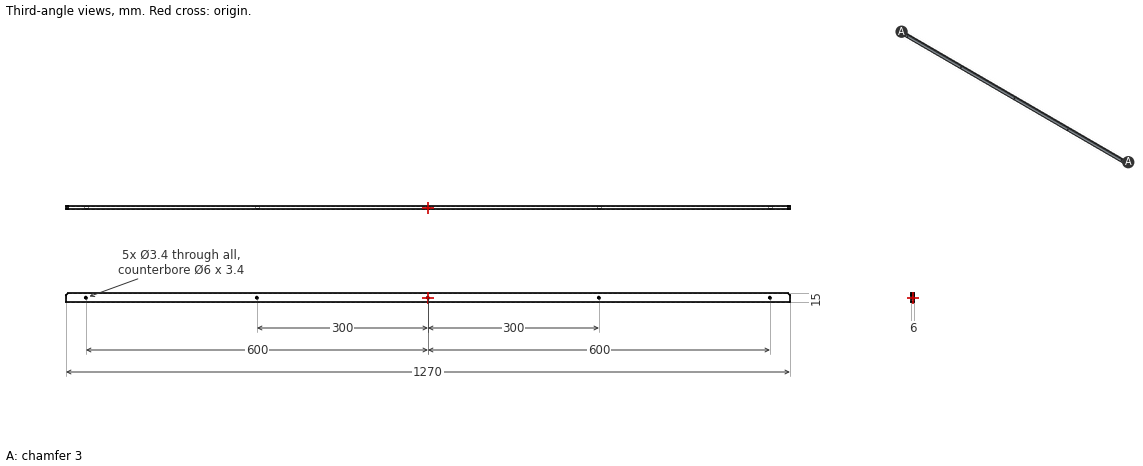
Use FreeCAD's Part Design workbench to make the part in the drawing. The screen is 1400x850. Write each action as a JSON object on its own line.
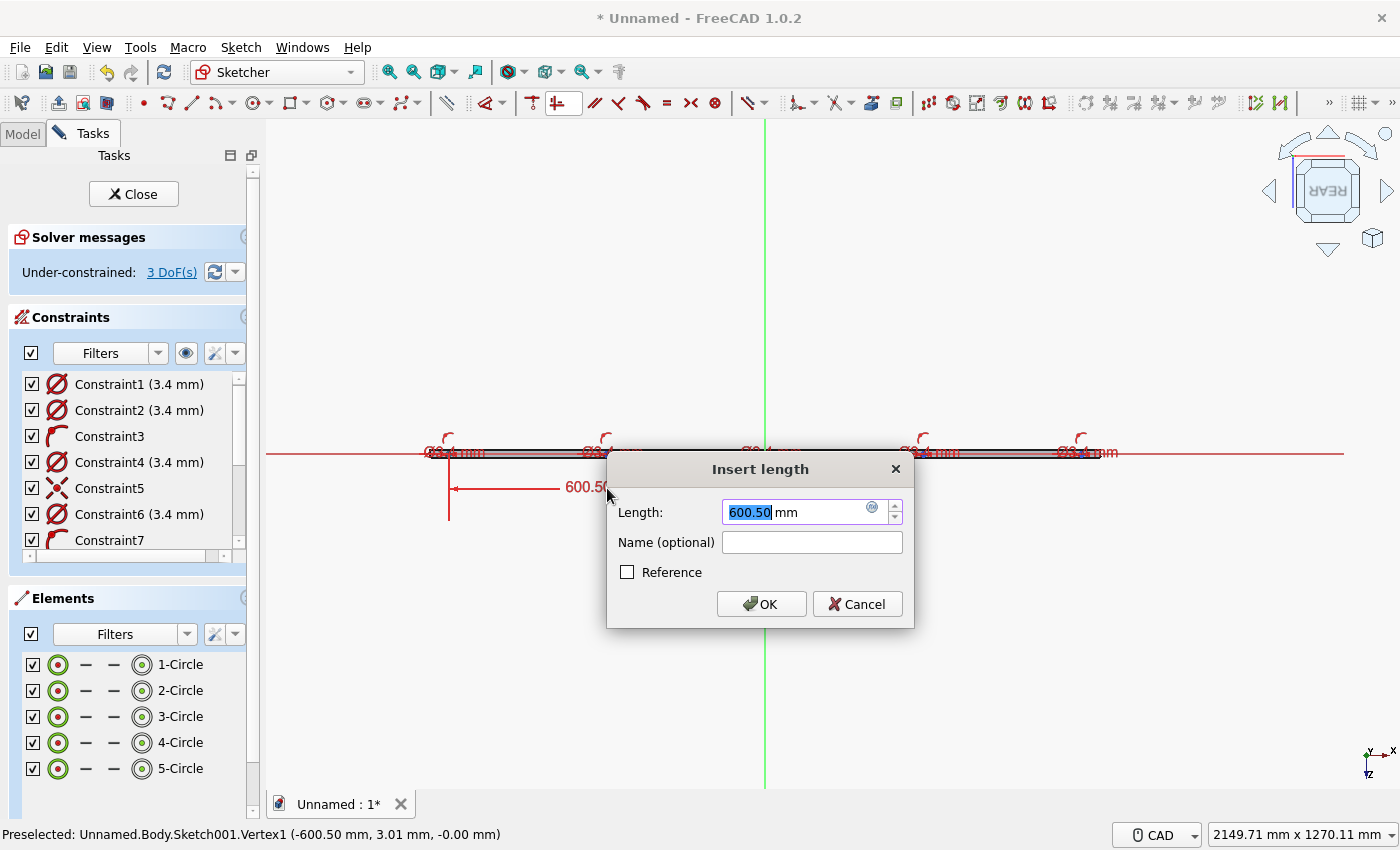
{"action": "type", "text": "600"}
{"action": "key", "text": "Return"}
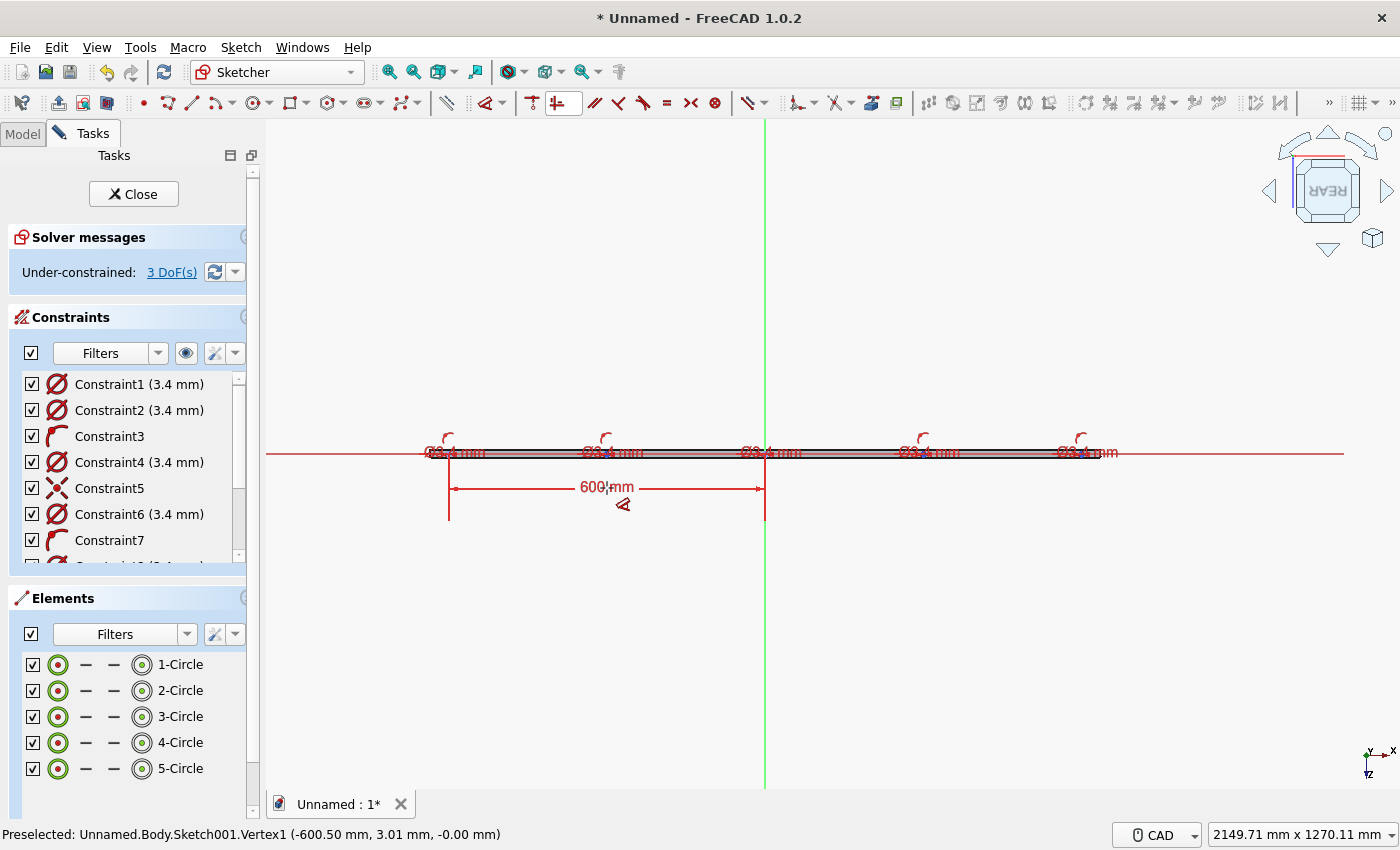
{"action": "left_click", "coordinate": [607, 454]}
{"action": "left_click", "coordinate": [686, 488]}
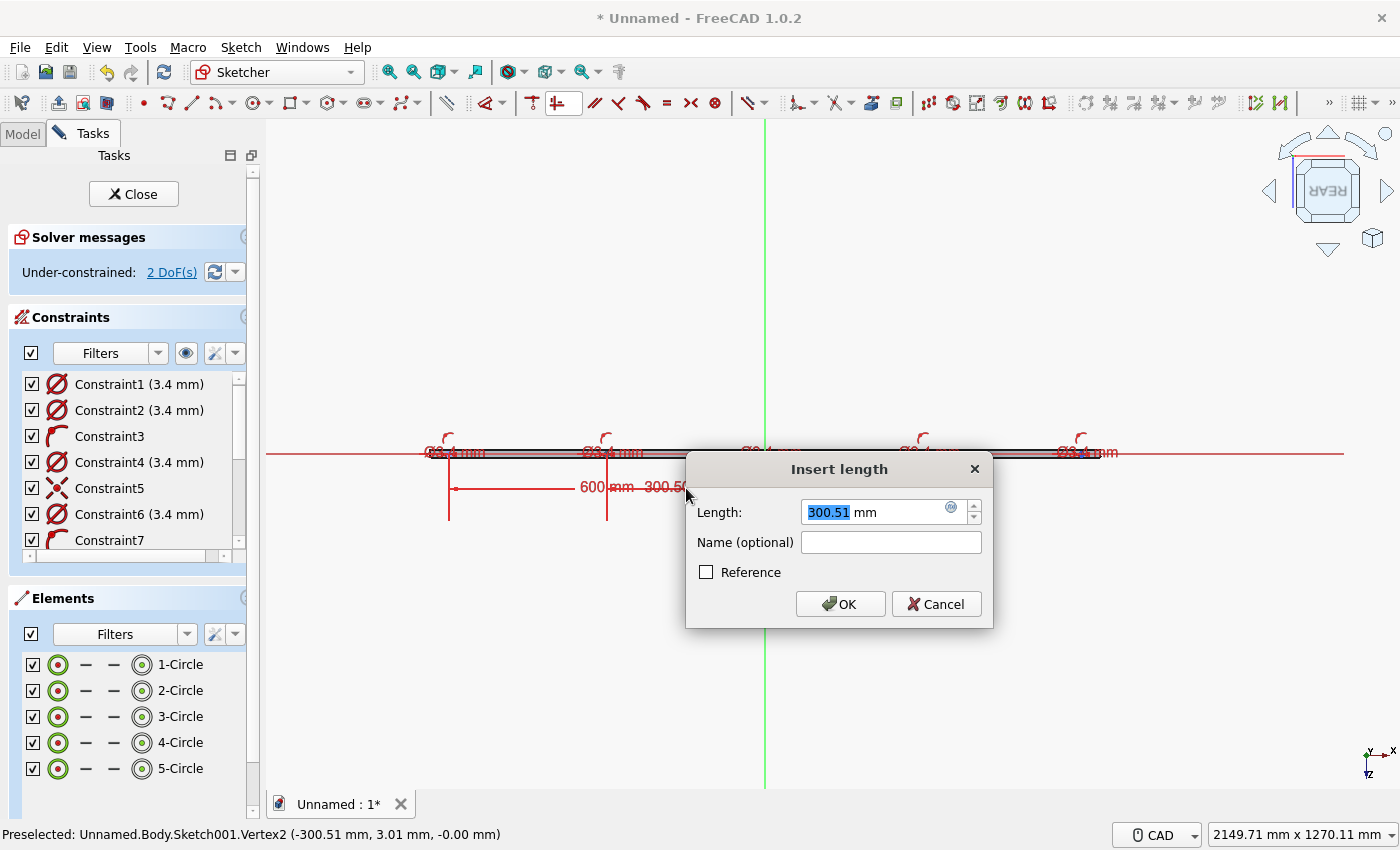
{"action": "type", "text": "300"}
{"action": "key", "text": "Return"}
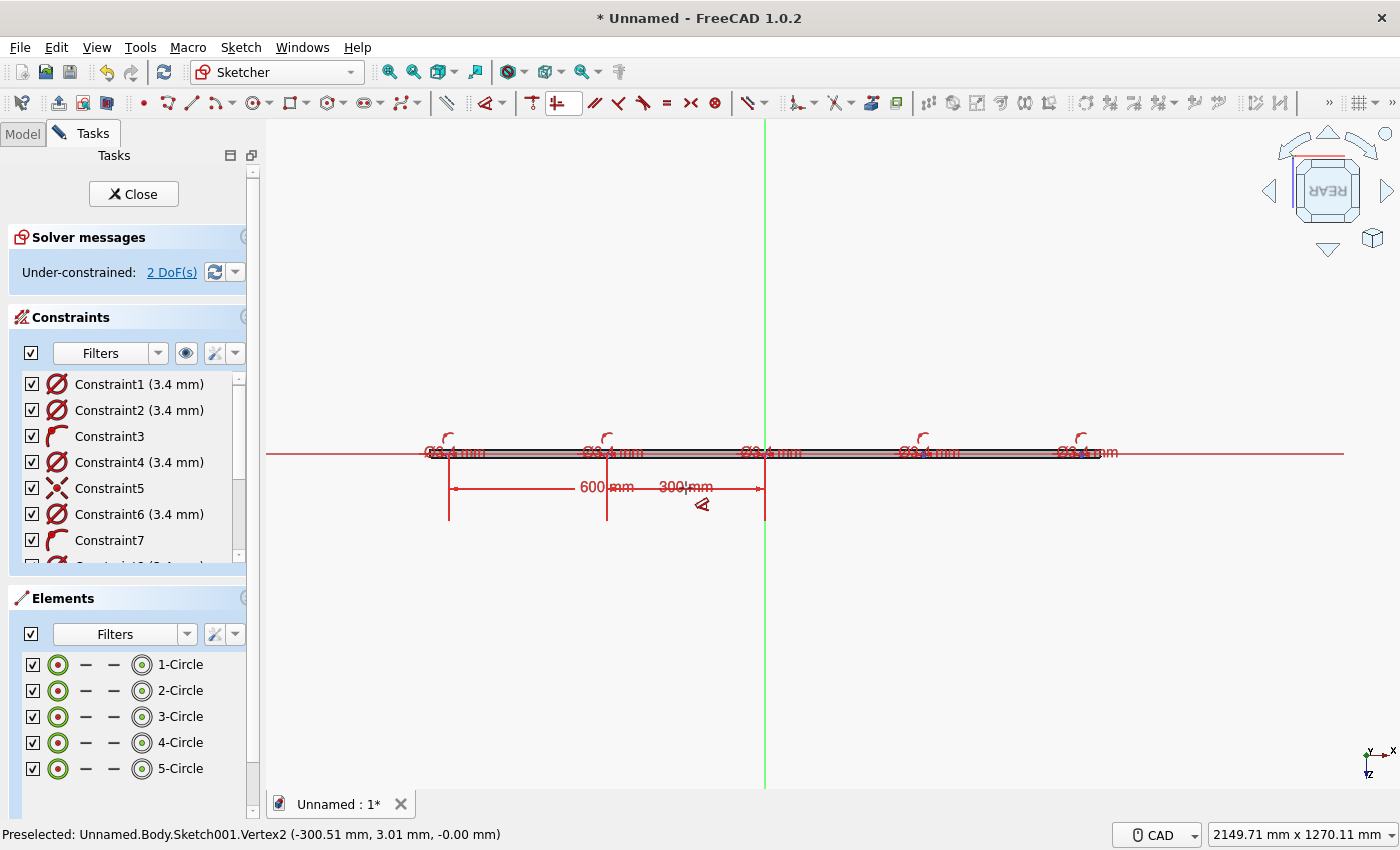
{"action": "left_click", "coordinate": [924, 454]}
{"action": "left_click", "coordinate": [845, 488]}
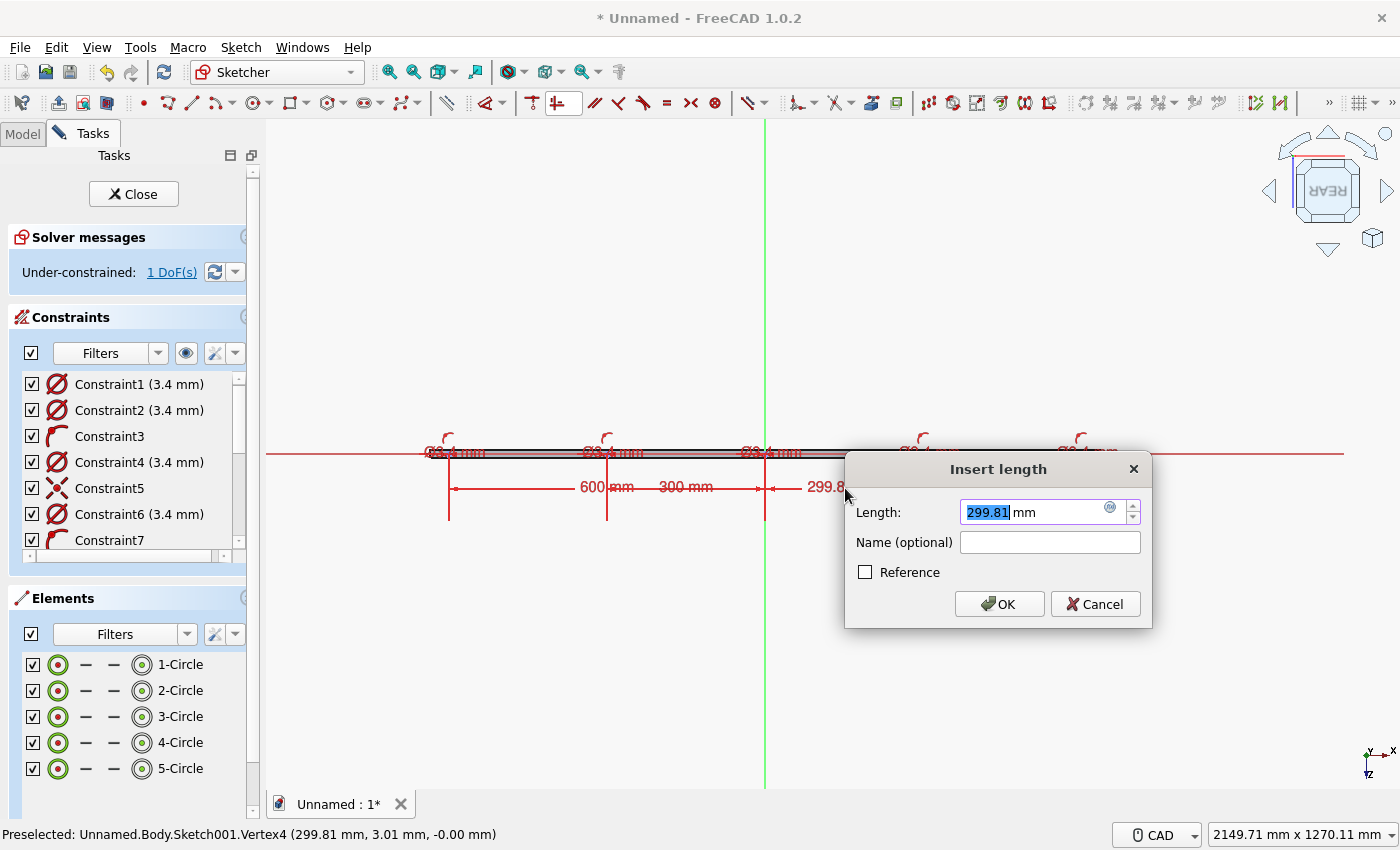
{"action": "type", "text": "300"}
{"action": "key", "text": "Return"}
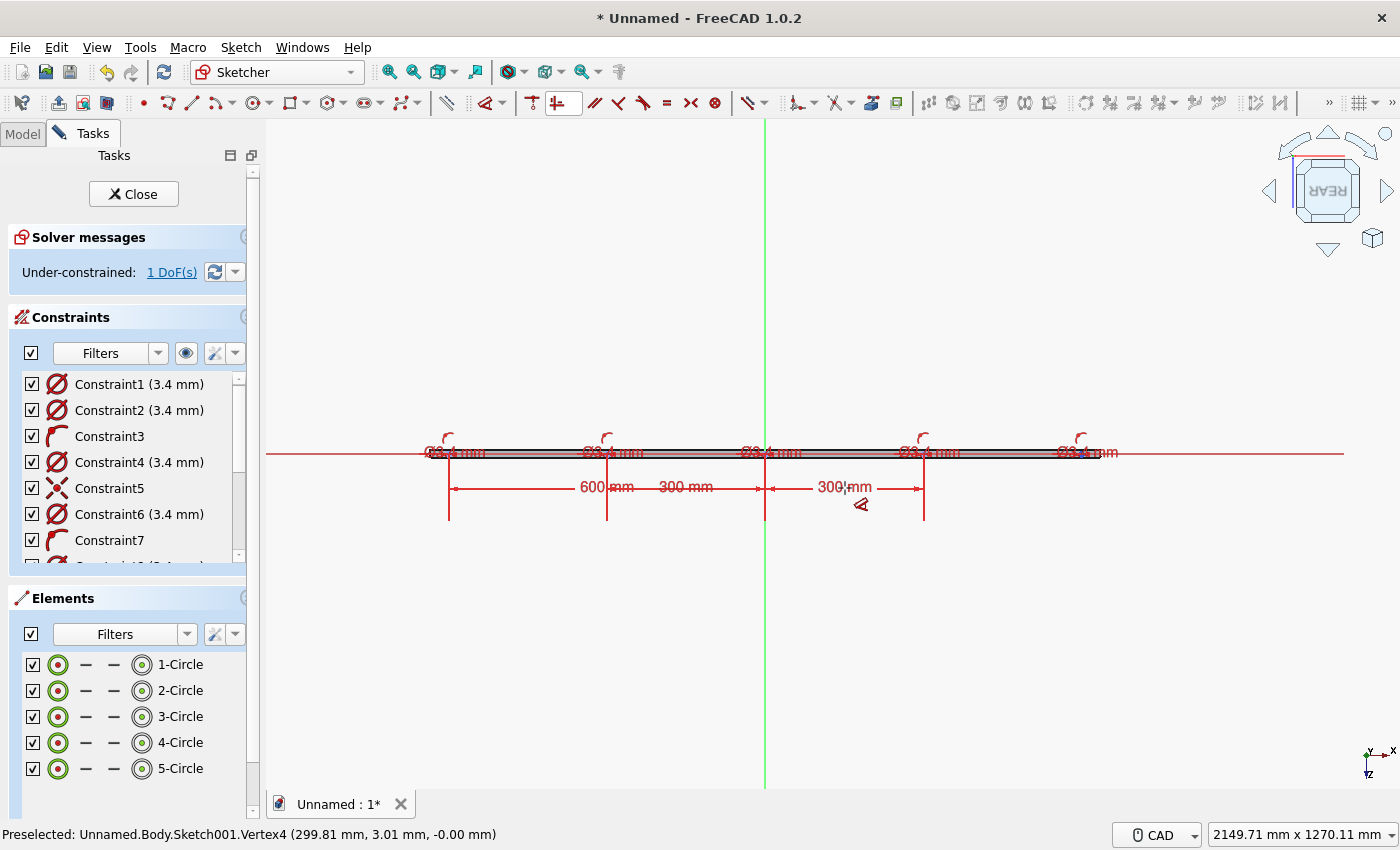
{"action": "left_click", "coordinate": [1082, 454]}
{"action": "left_click", "coordinate": [924, 488]}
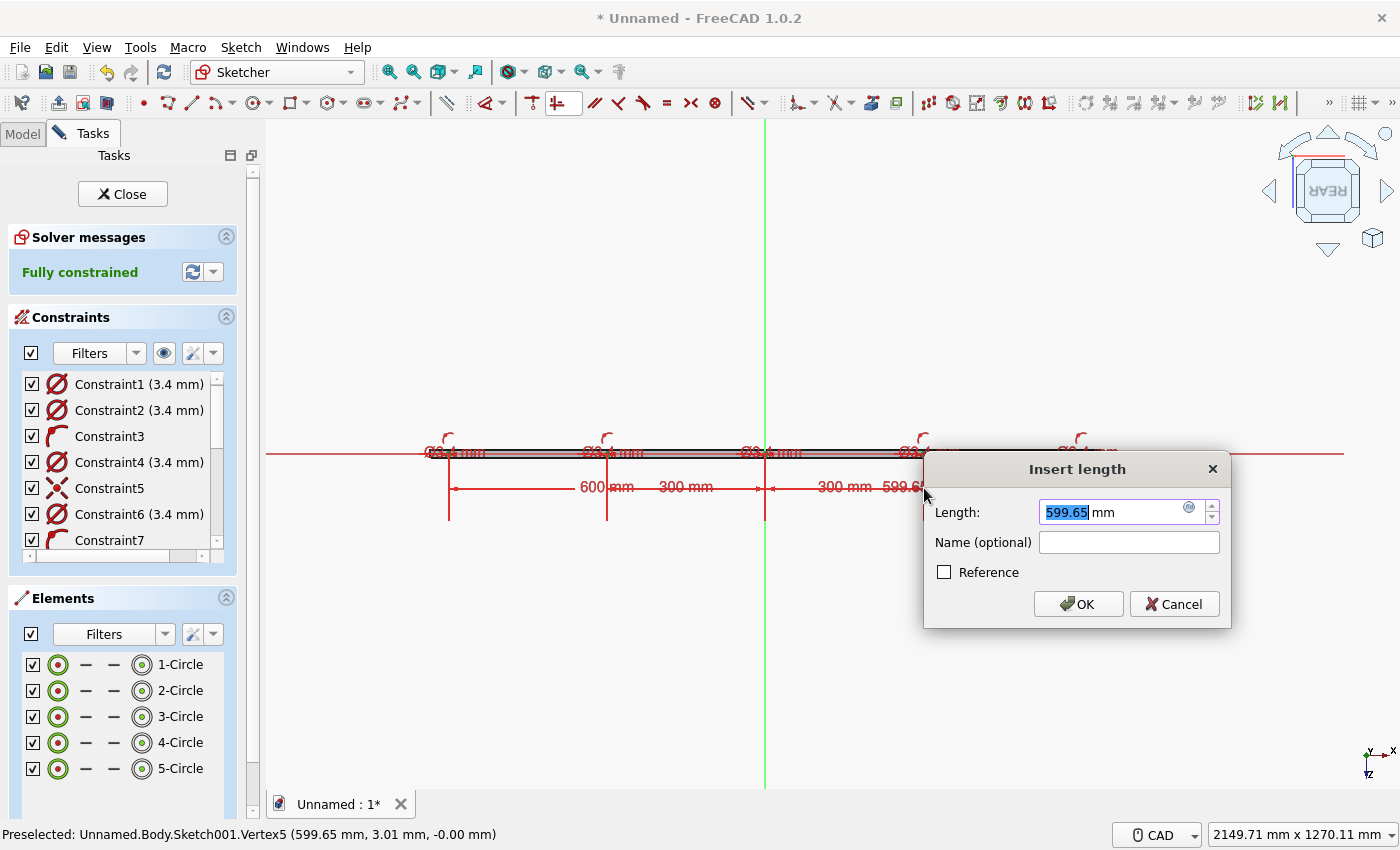
{"action": "type", "text": "600"}
{"action": "key", "text": "Return"}
{"action": "key", "text": "Escape"}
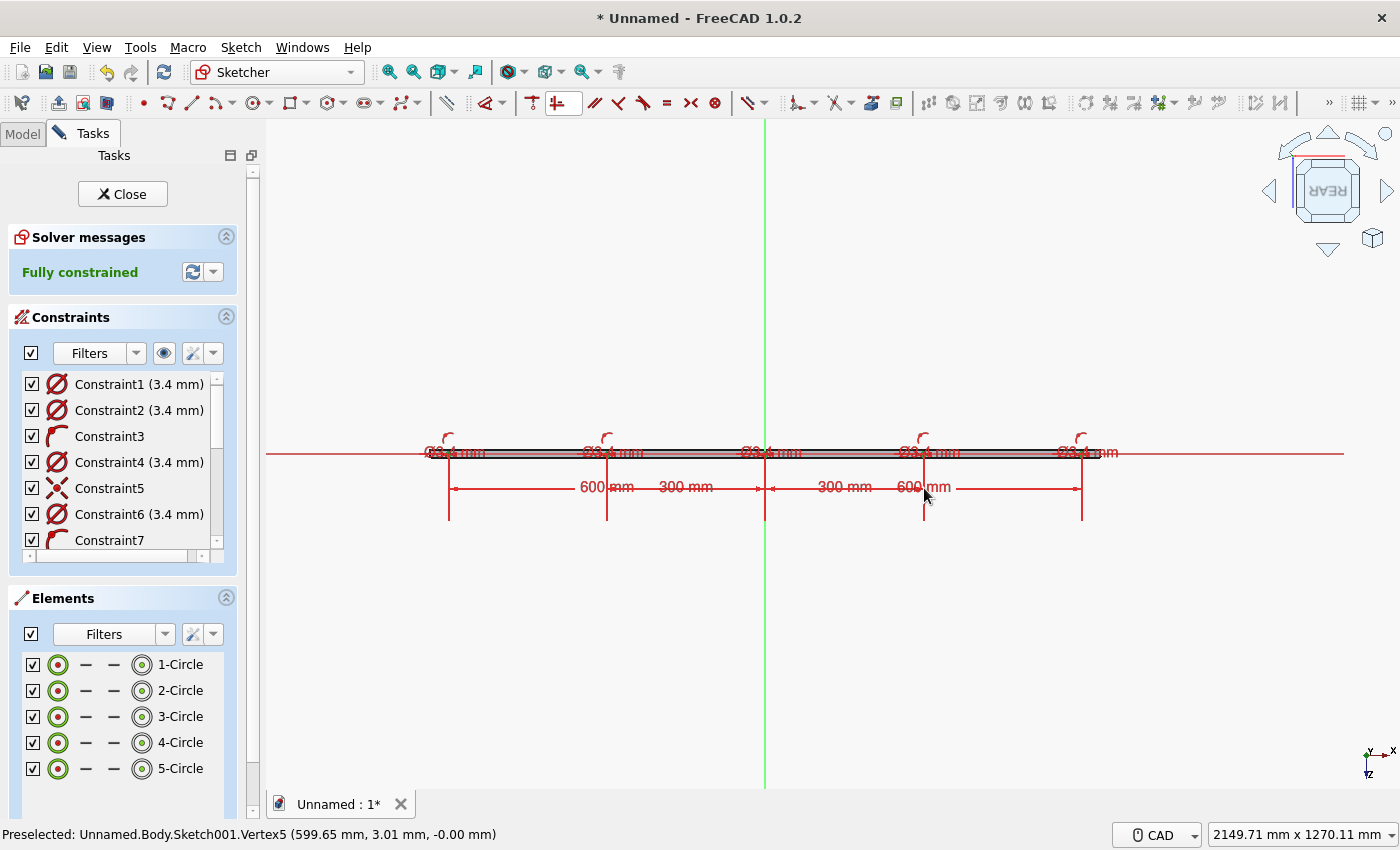
{"action": "left_click", "coordinate": [123, 194]}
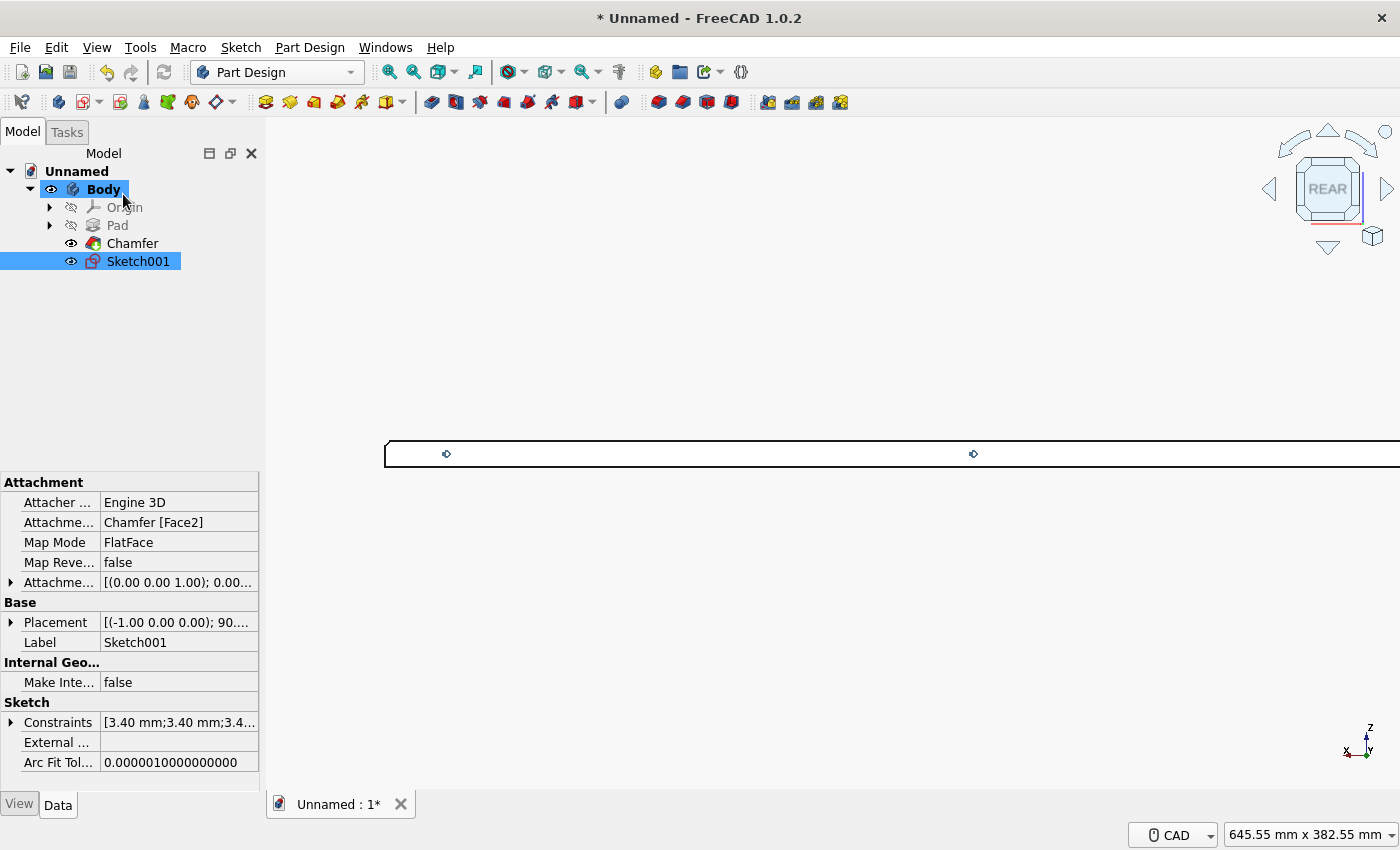
{"action": "left_click", "coordinate": [456, 102]}